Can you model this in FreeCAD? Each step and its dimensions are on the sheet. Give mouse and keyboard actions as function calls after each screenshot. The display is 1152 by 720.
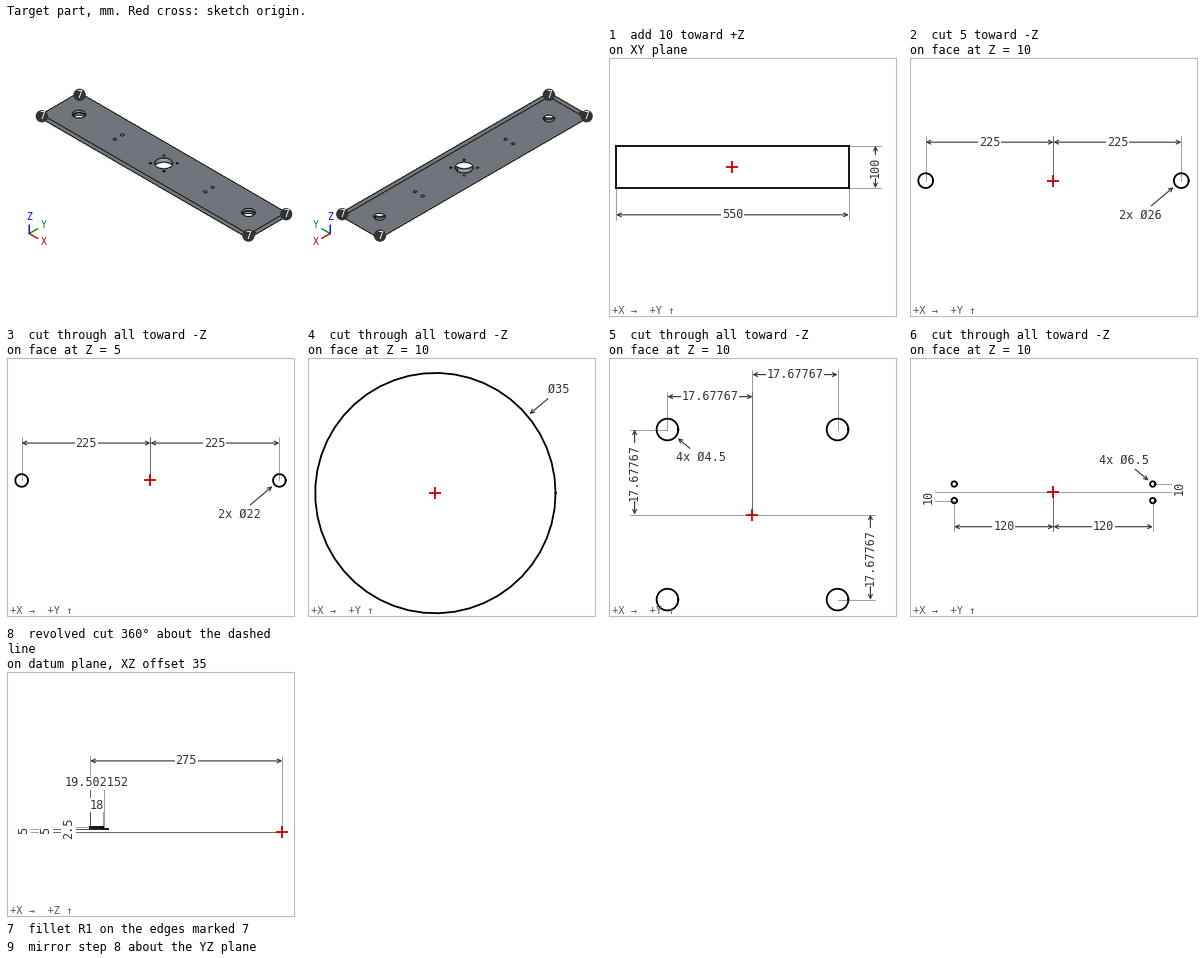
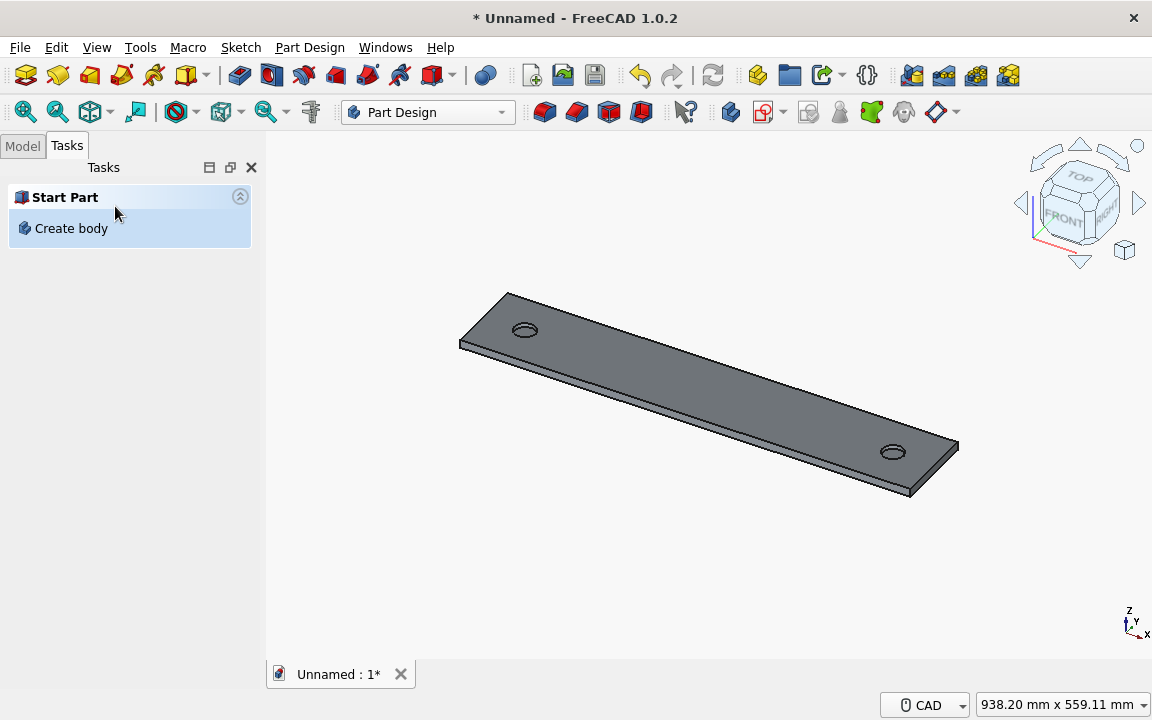
key(0)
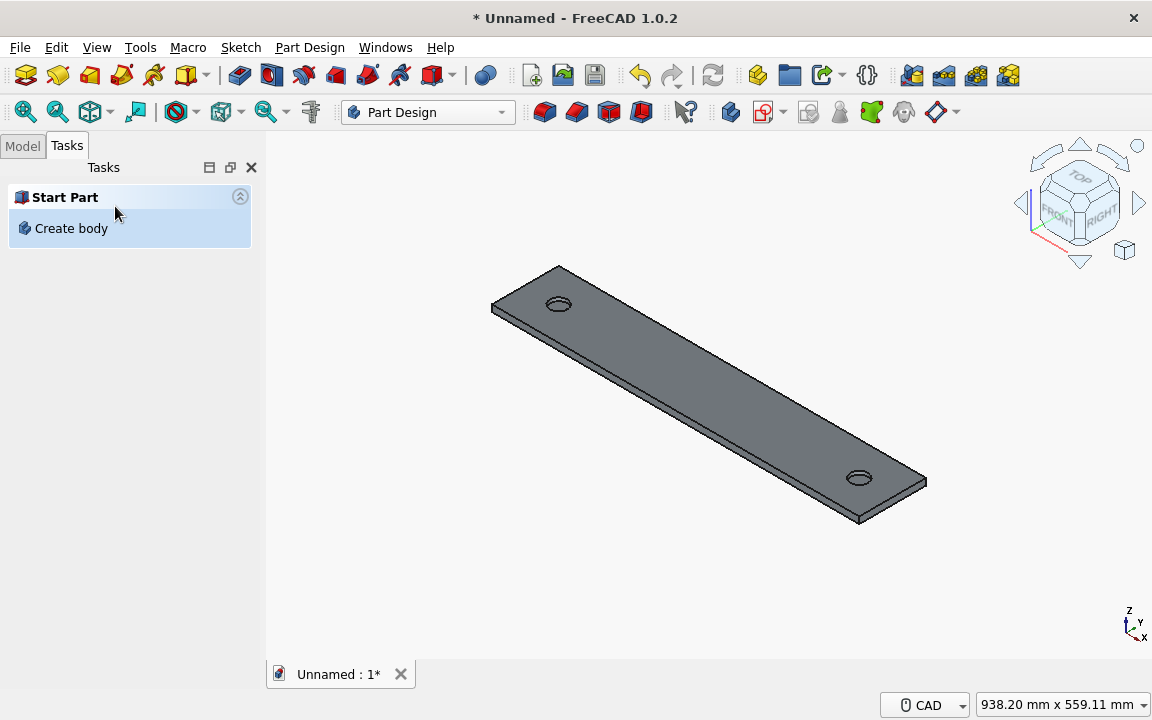
key(2)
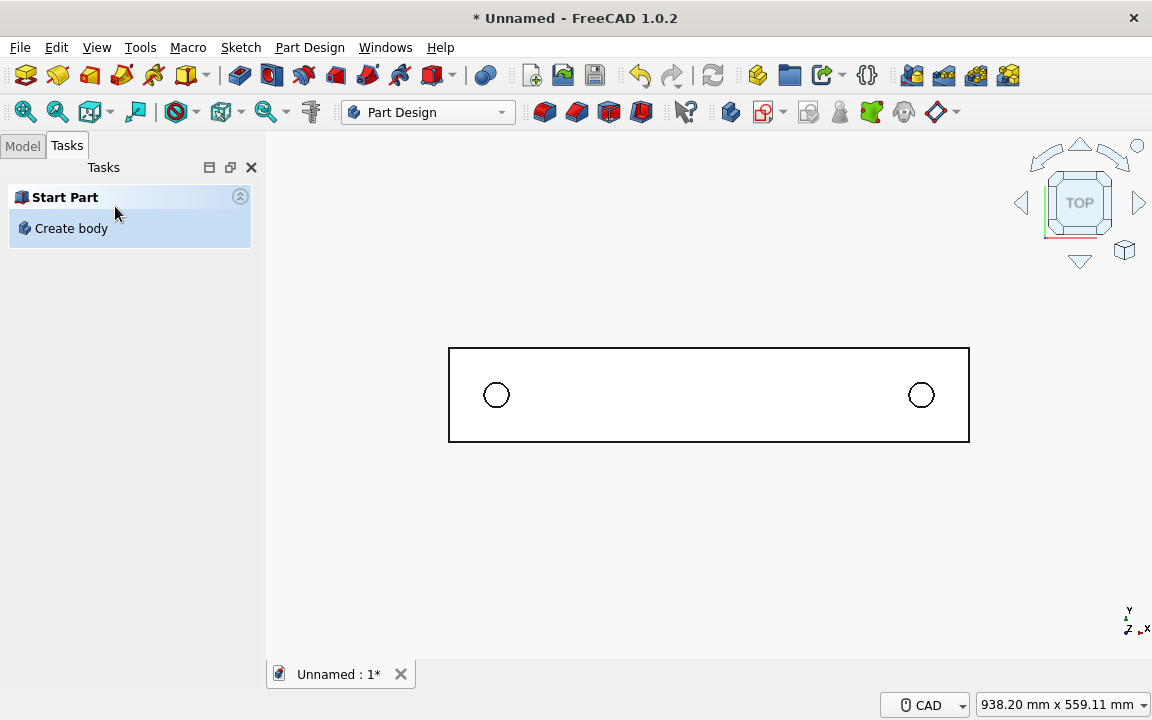
click(497, 394)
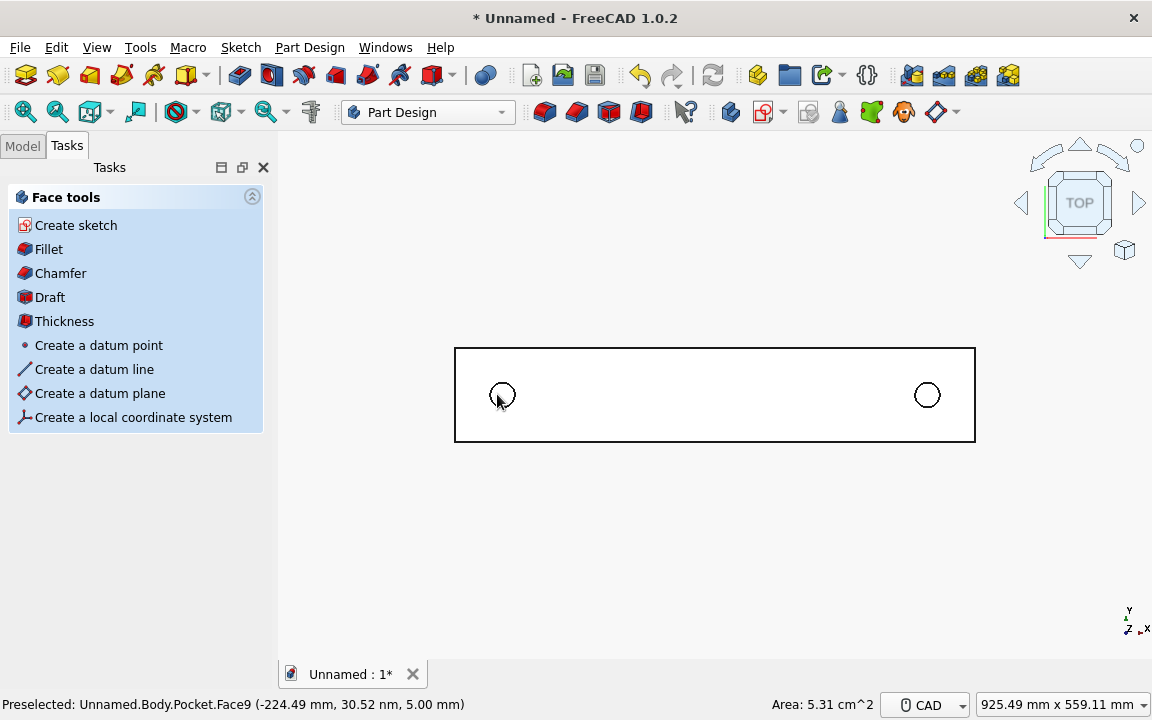
click(764, 112)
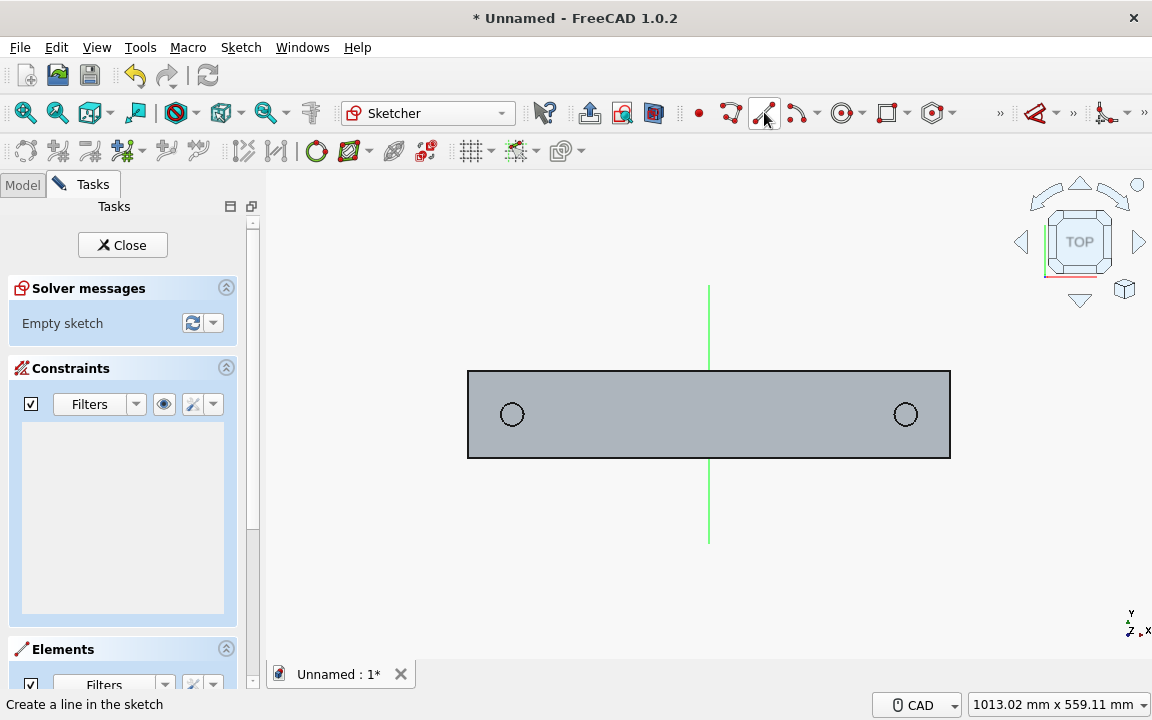
click(654, 114)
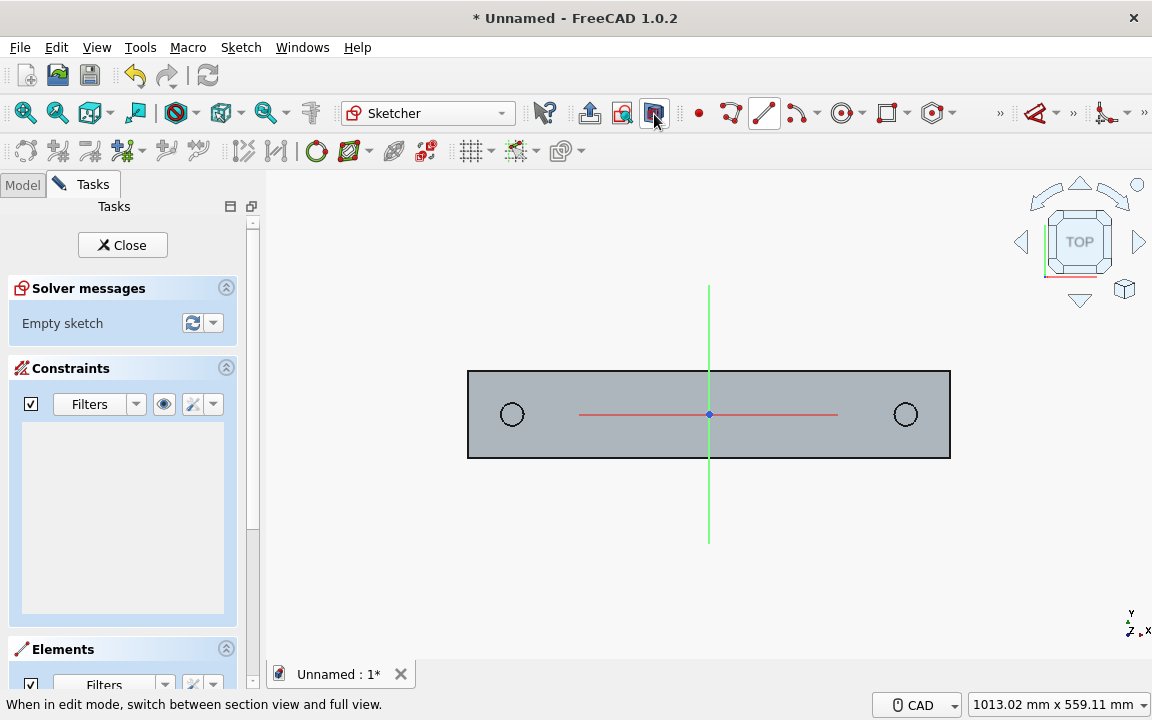
click(842, 114)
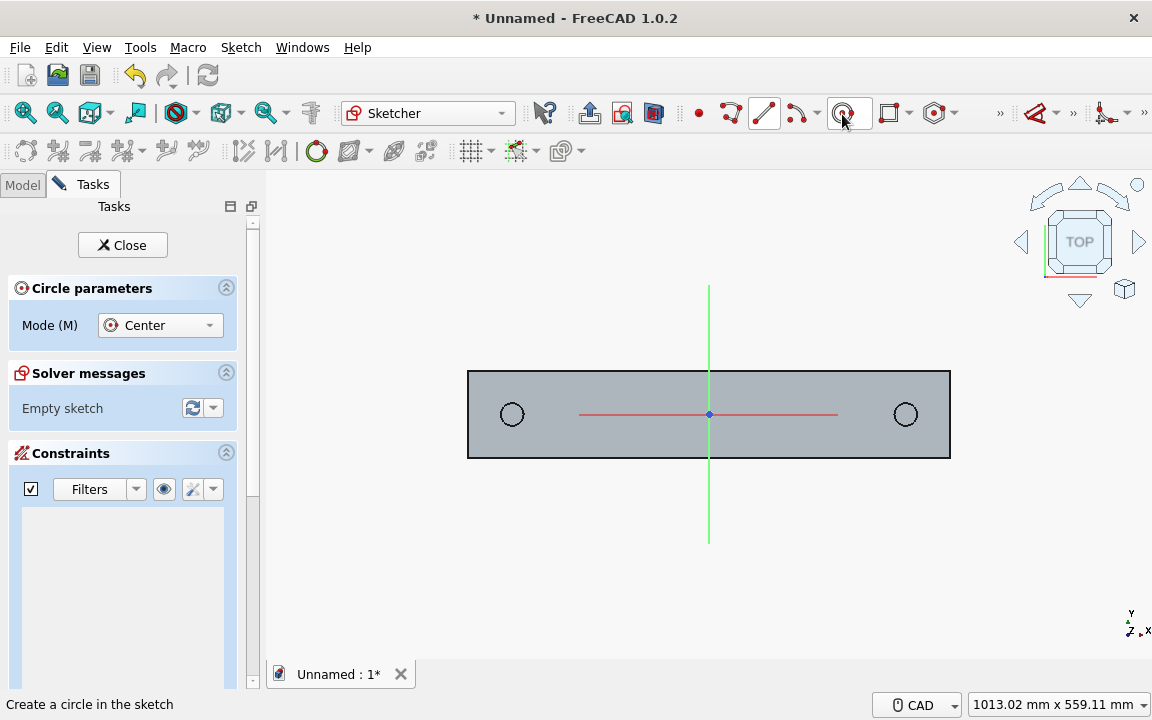
scroll(906, 415, up, 5)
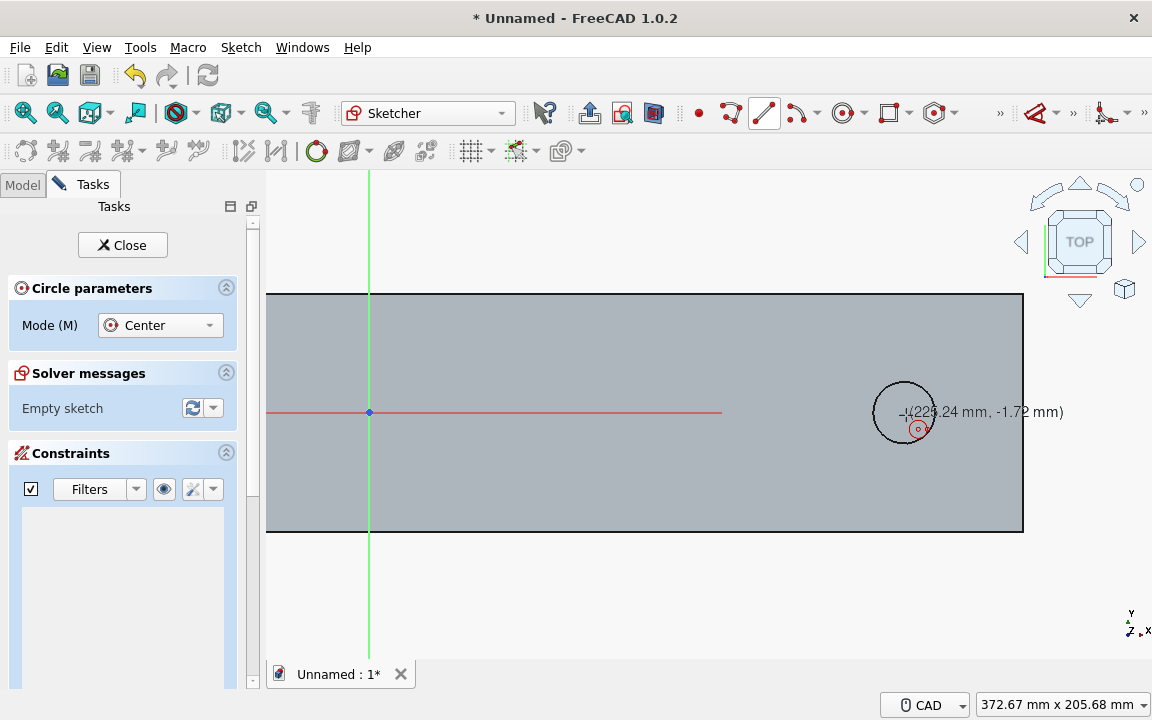
click(904, 413)
move(923, 394)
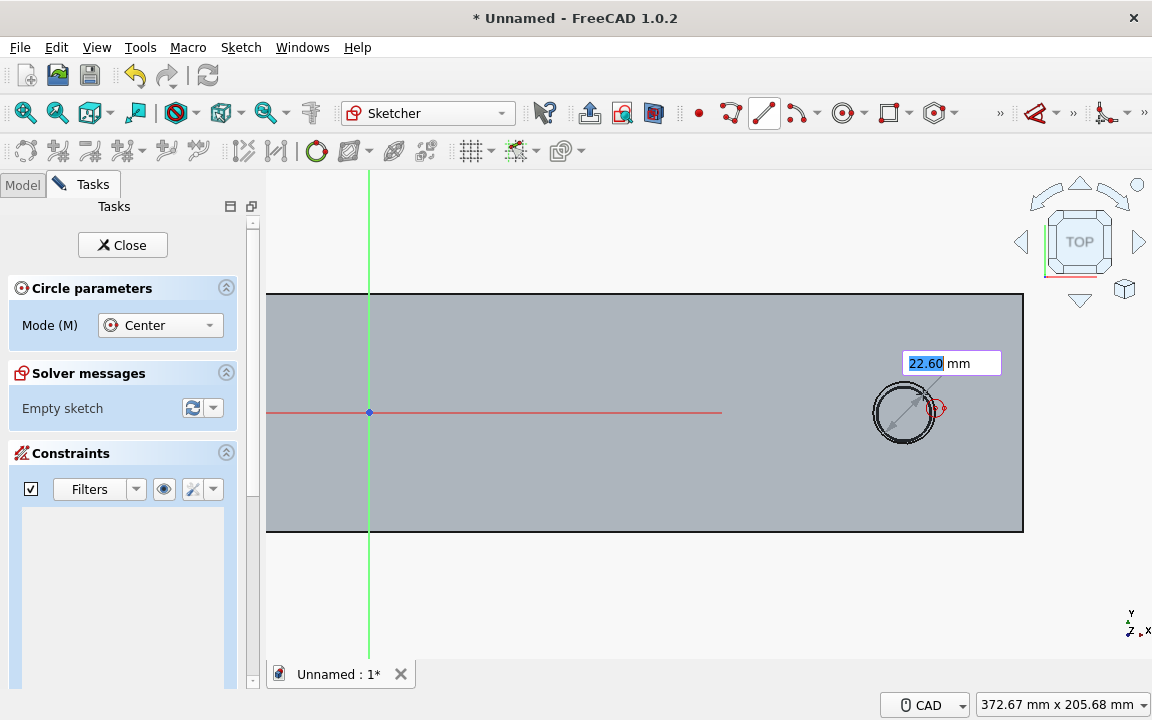
text(22)
key(Return)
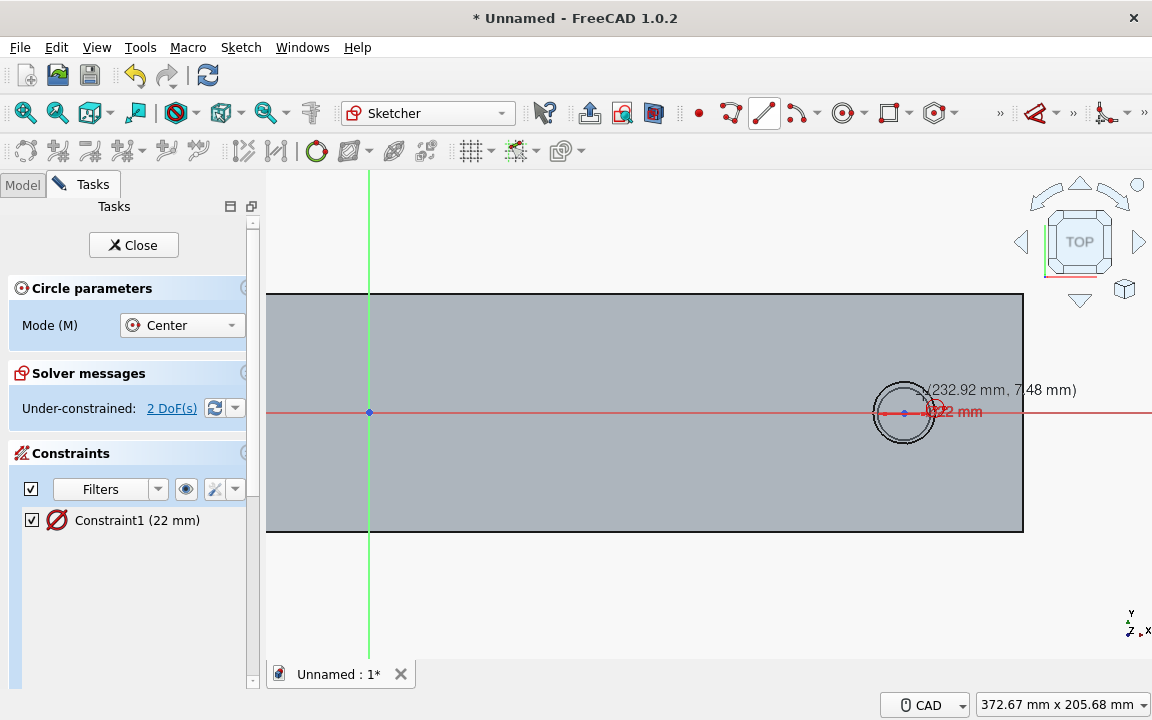
scroll(862, 416, down, 4)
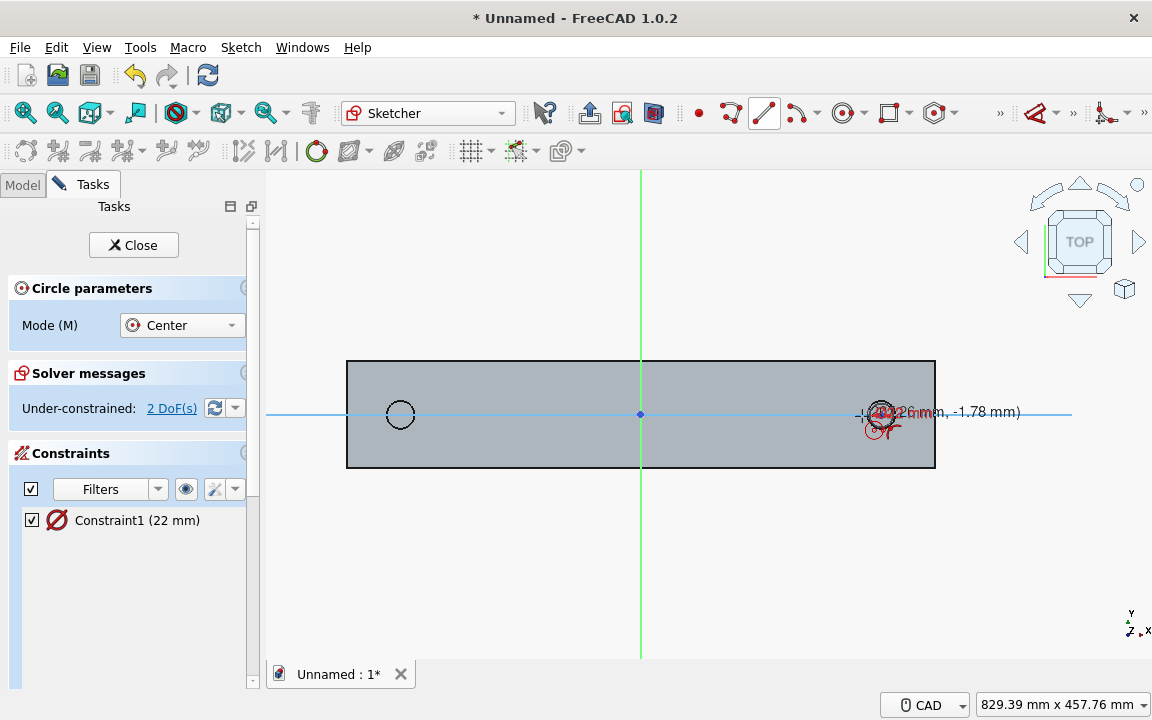
scroll(401, 415, up, 4)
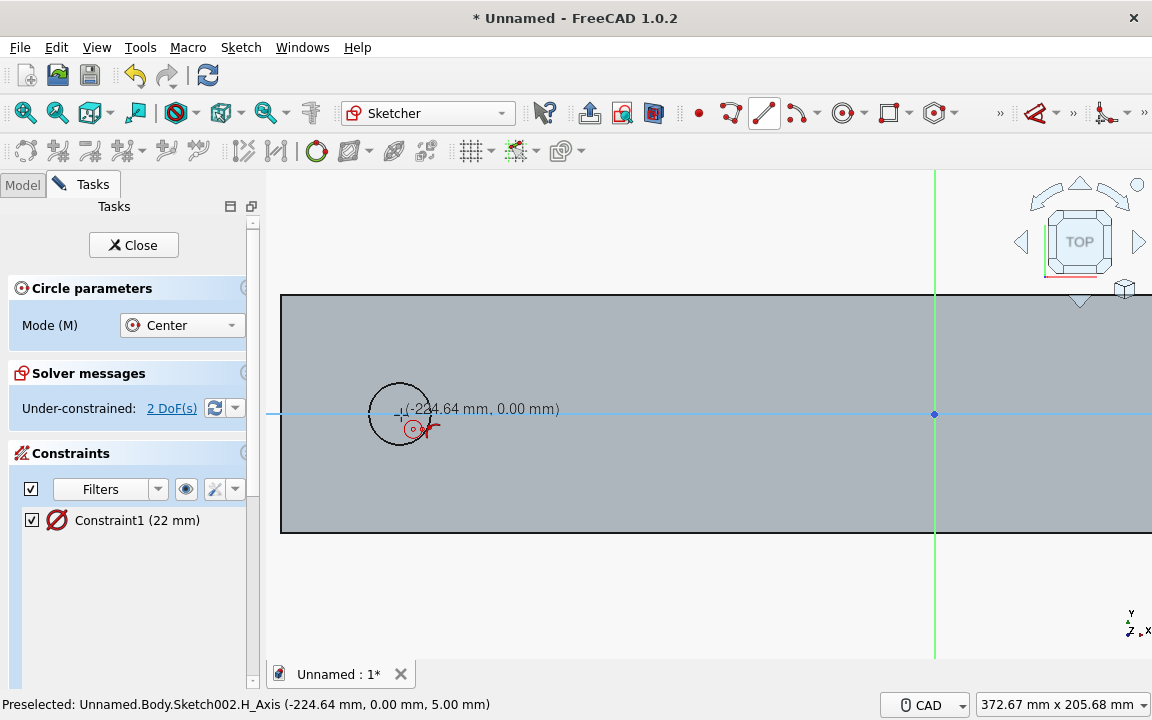
click(400, 414)
move(418, 396)